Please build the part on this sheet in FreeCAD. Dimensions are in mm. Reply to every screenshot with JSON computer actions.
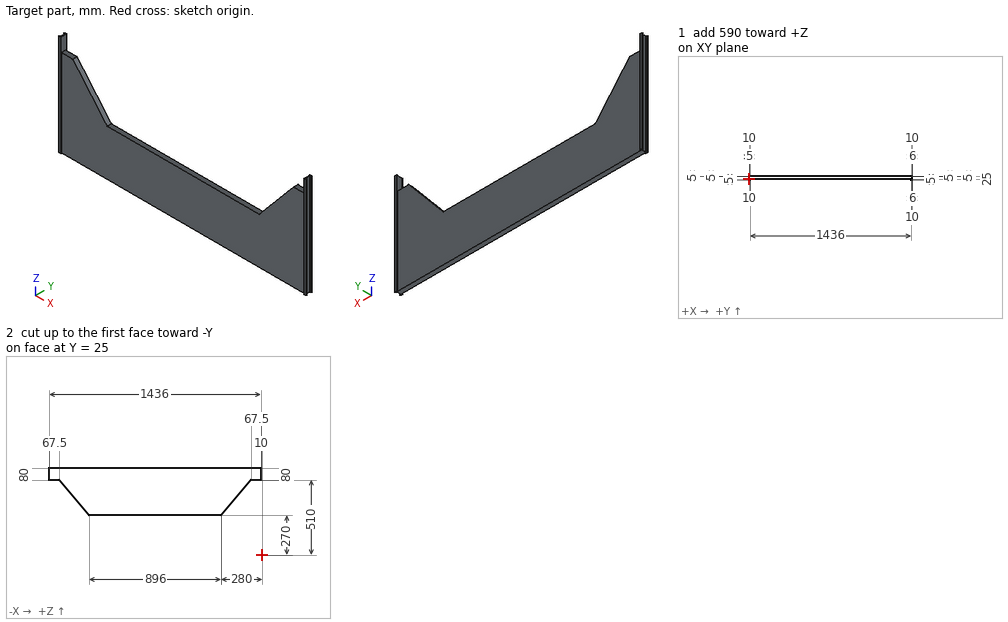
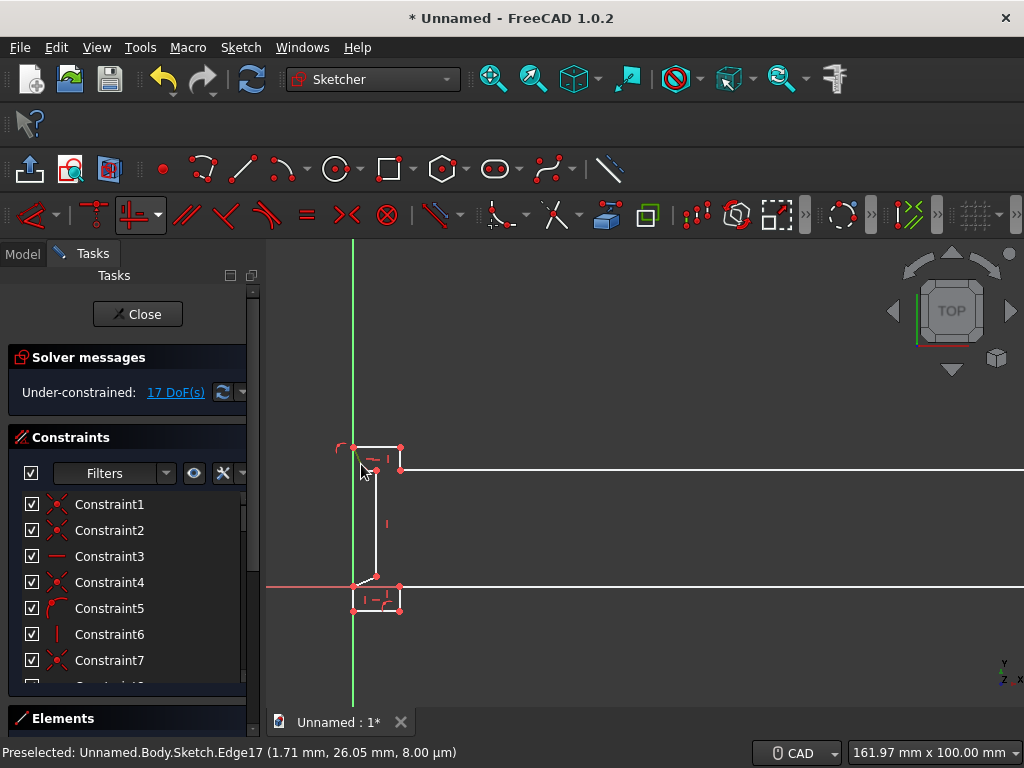
{"action": "key", "text": "v"}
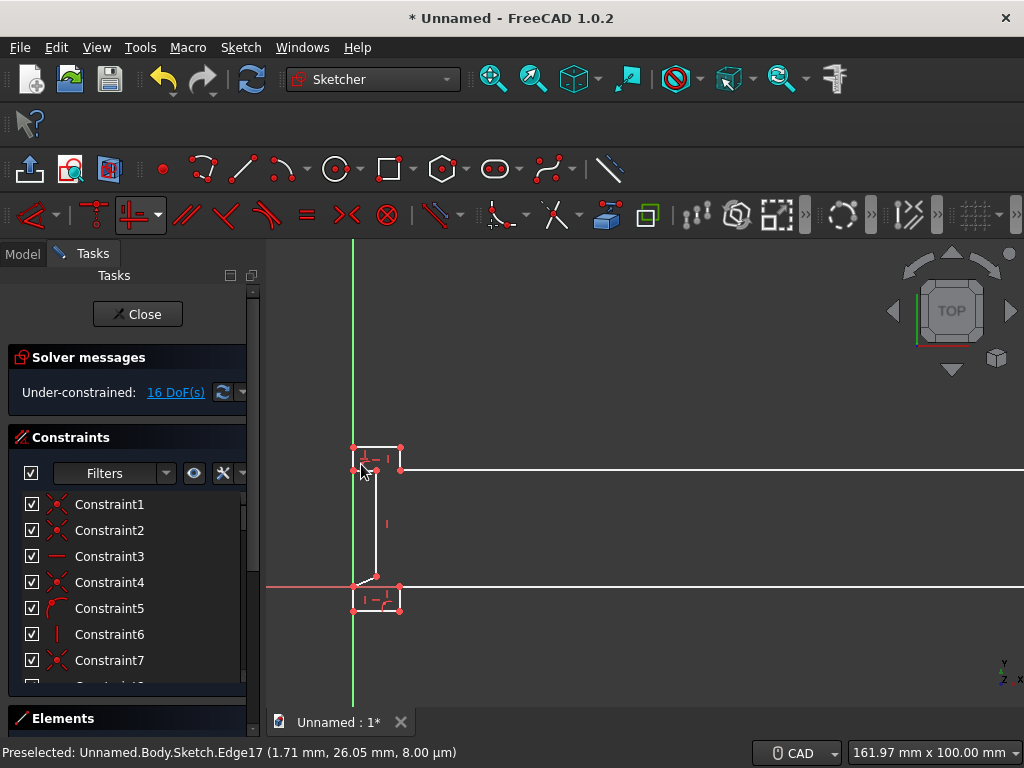
{"action": "left_click", "coordinate": [363, 583]}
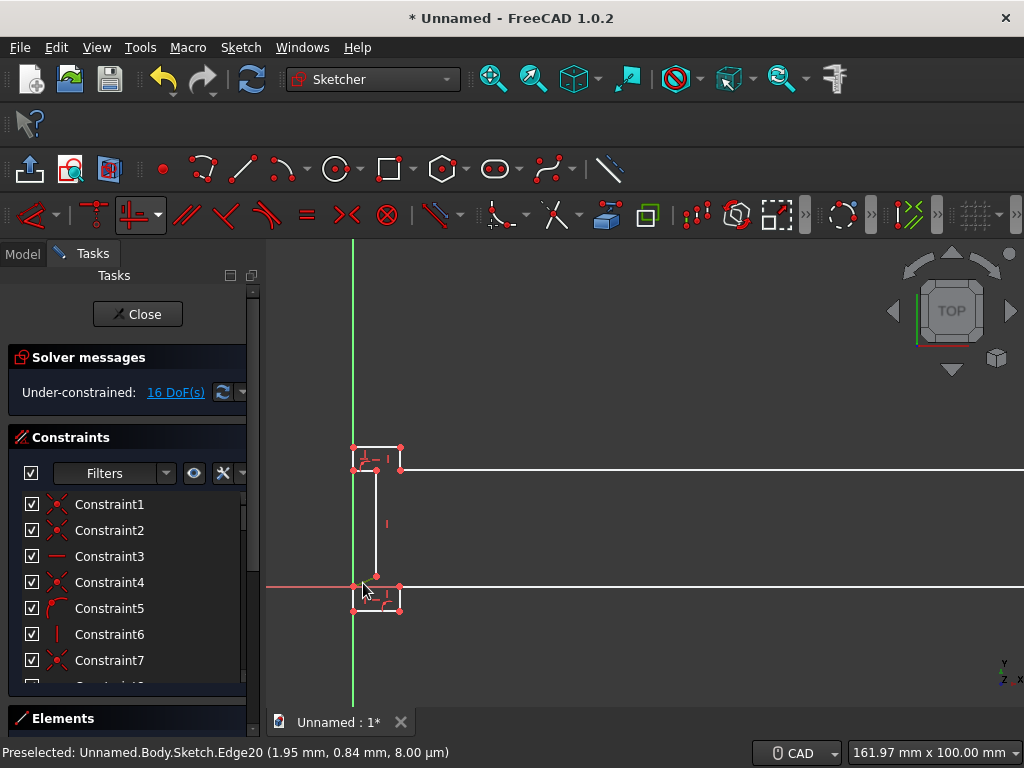
{"action": "key", "text": "h"}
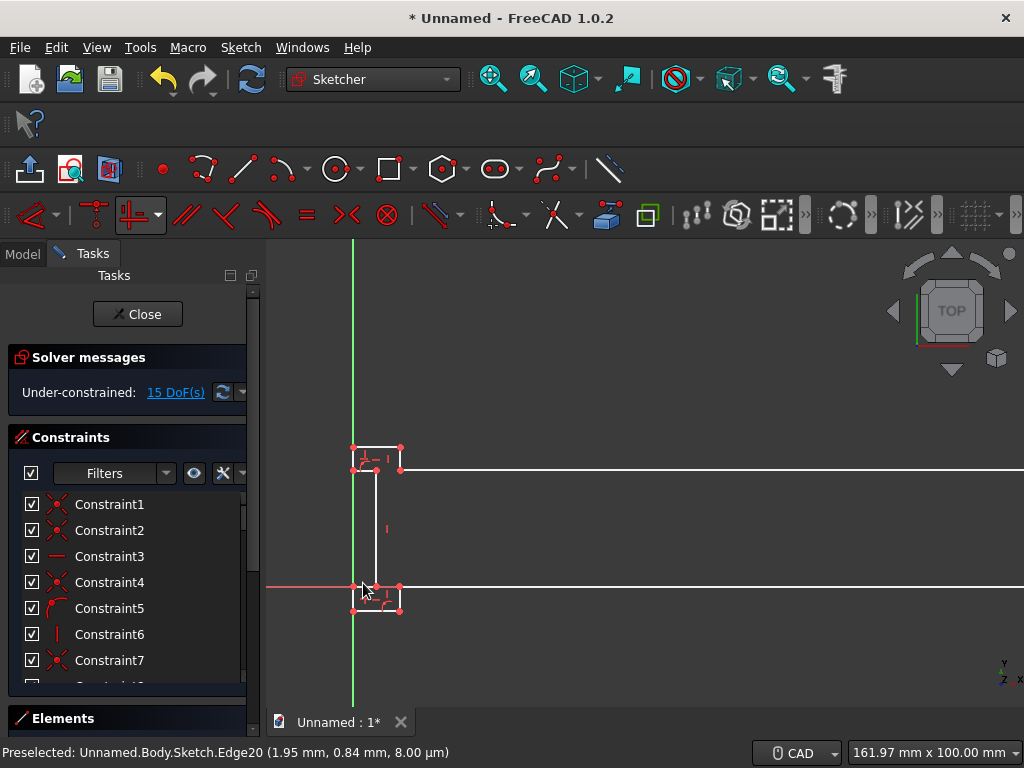
{"action": "key", "text": "d"}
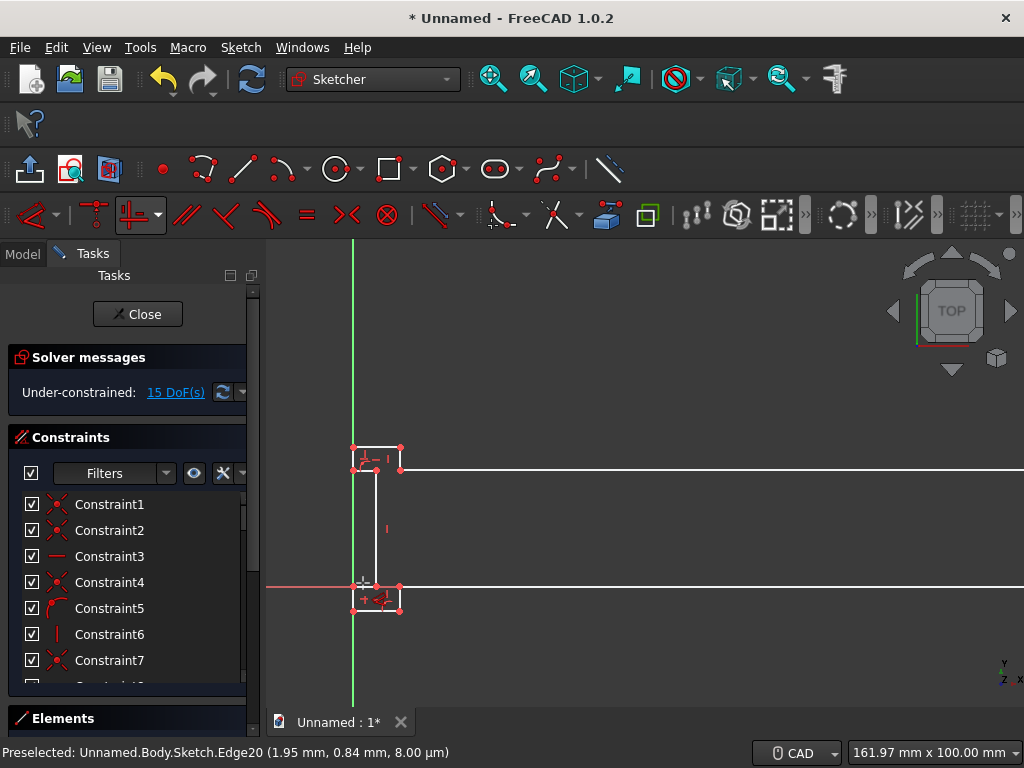
{"action": "scroll", "coordinate": [353, 597], "scroll_direction": "up", "scroll_amount": 3}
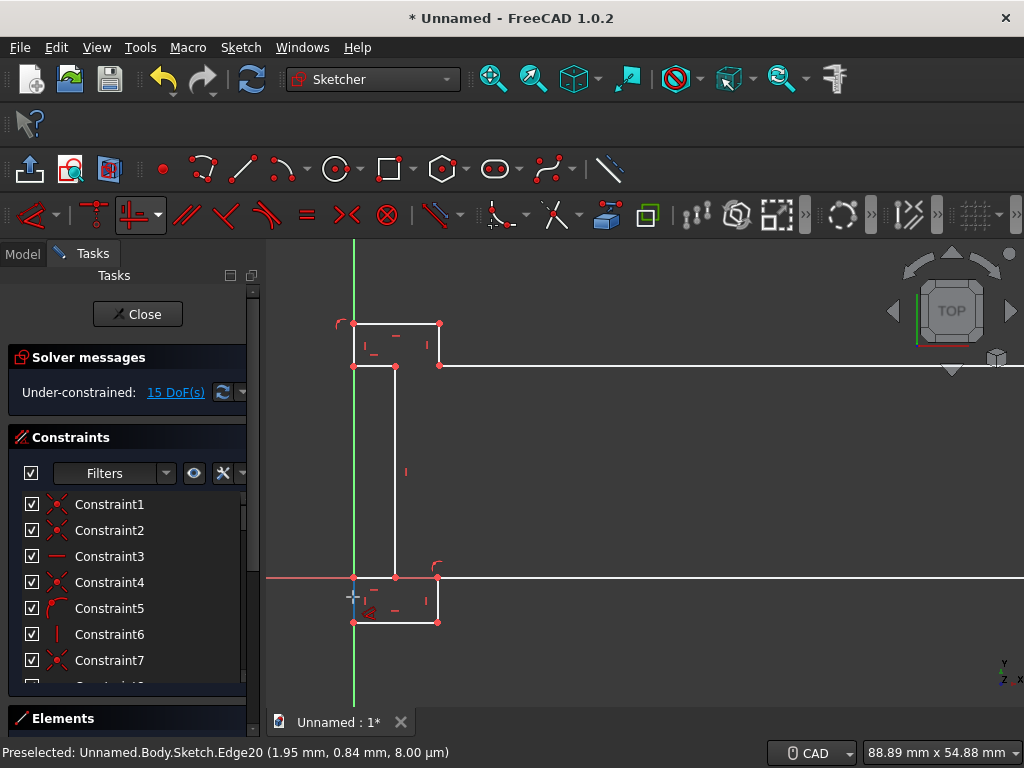
{"action": "left_click", "coordinate": [354, 596]}
{"action": "left_click", "coordinate": [320, 600]}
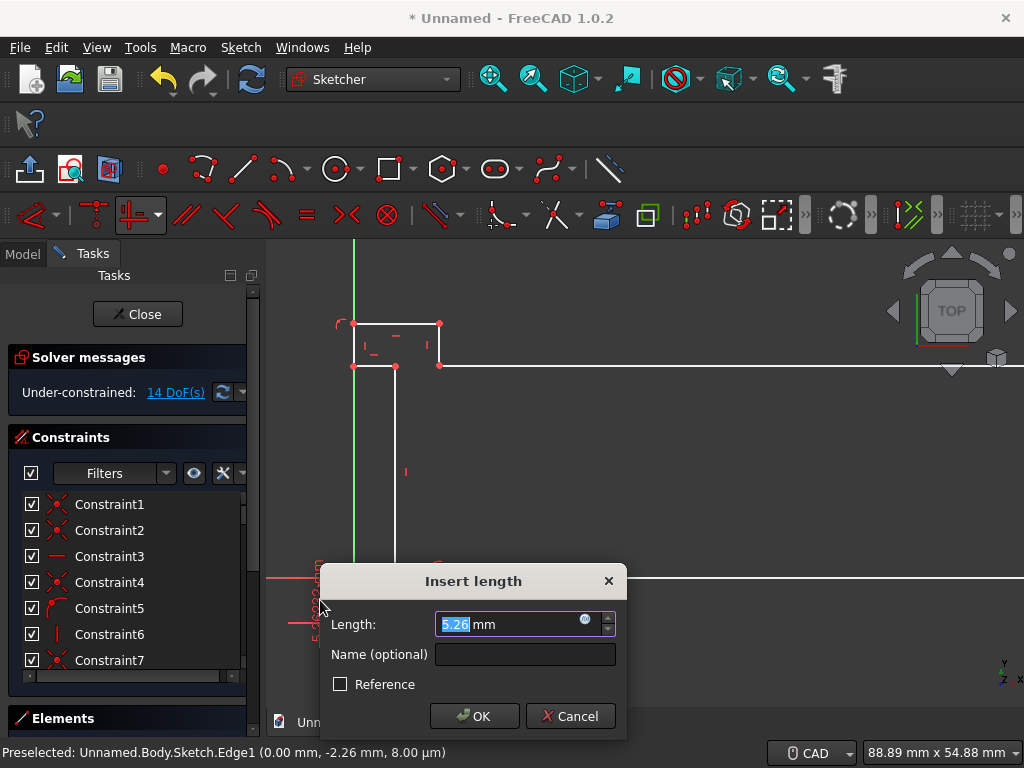
{"action": "type", "text": "5"}
{"action": "key", "text": "Return"}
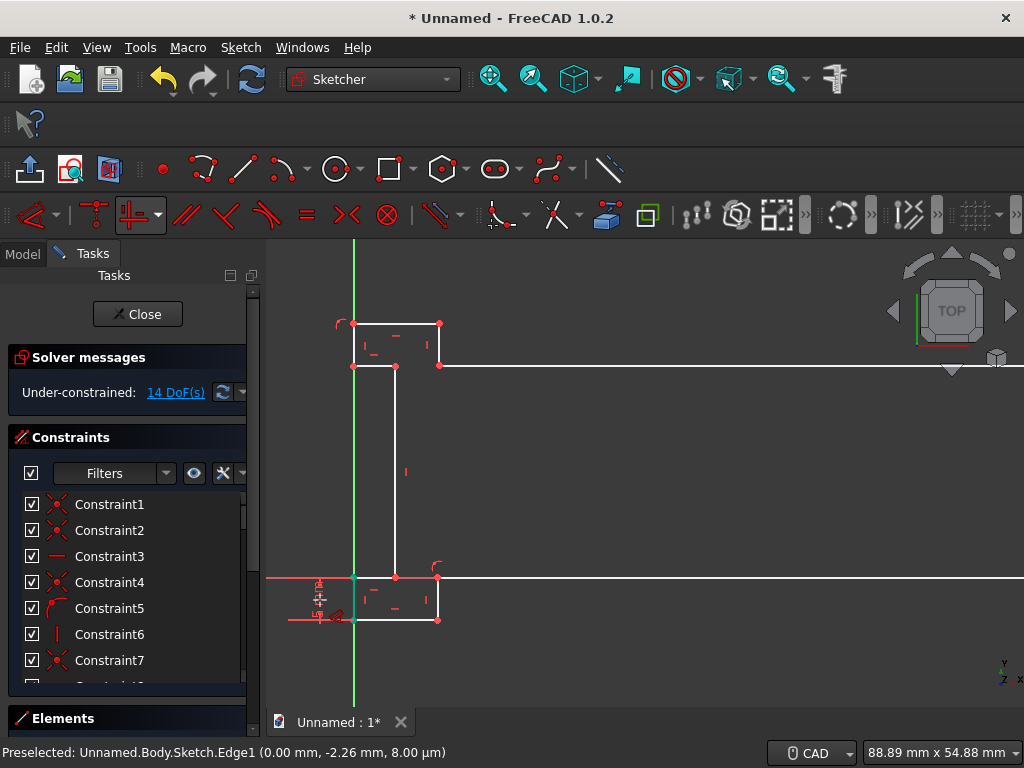
{"action": "scroll", "coordinate": [322, 473], "scroll_direction": "down", "scroll_amount": 16}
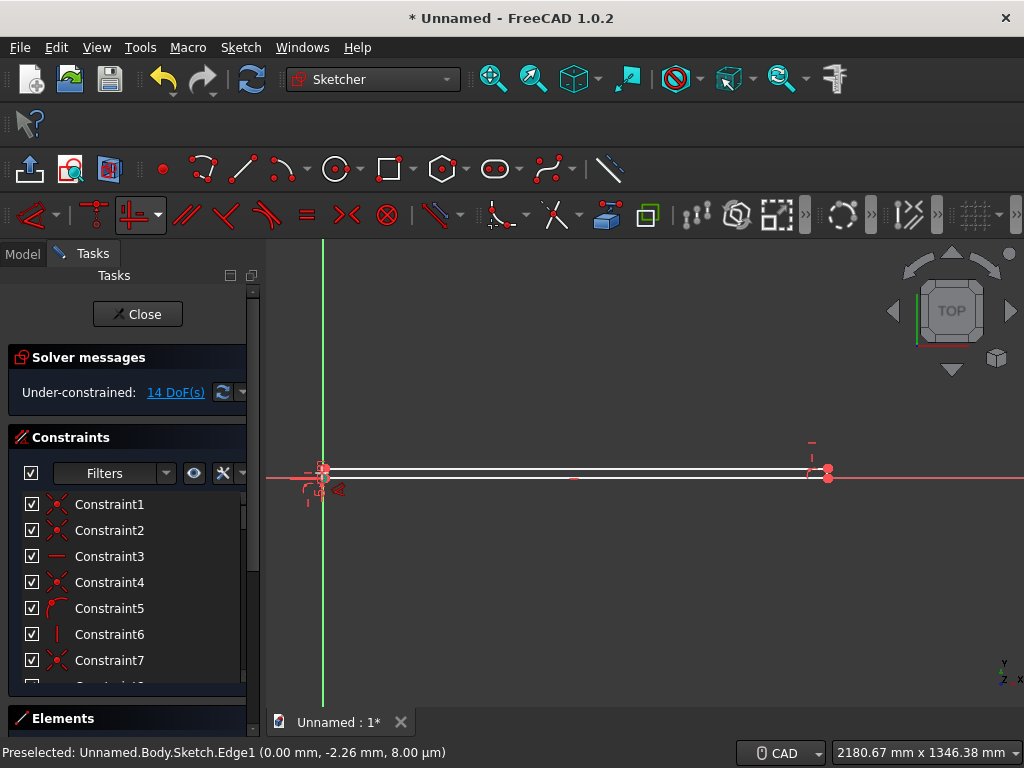
{"action": "scroll", "coordinate": [827, 478], "scroll_direction": "up", "scroll_amount": 16}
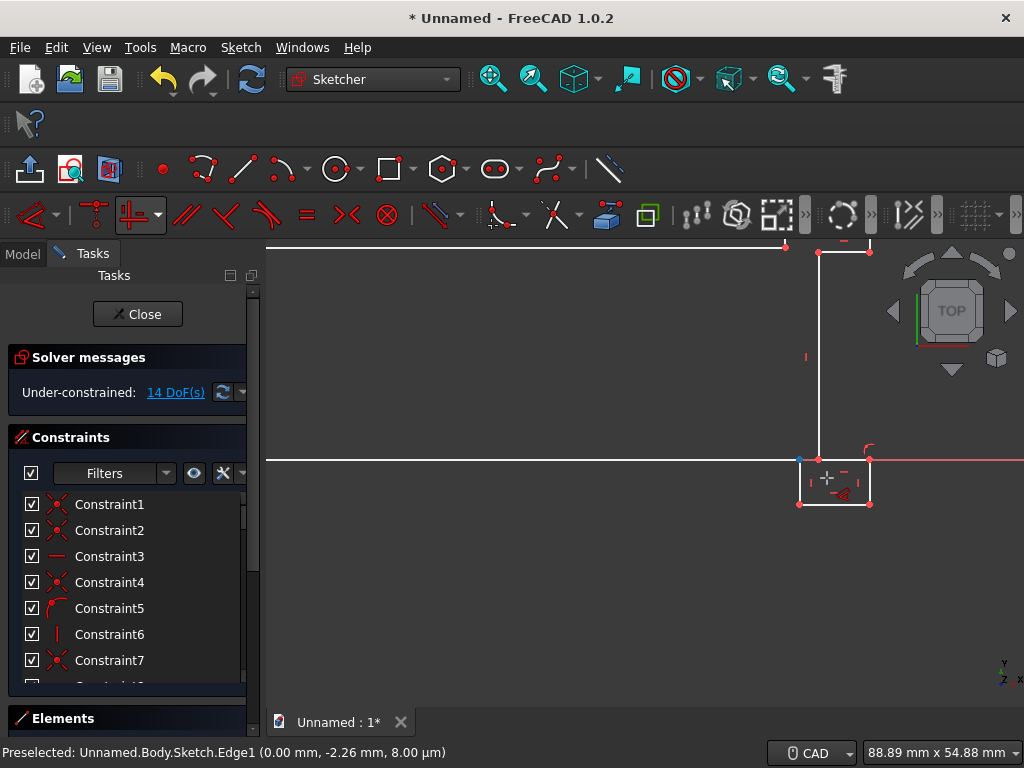
{"action": "left_click", "coordinate": [800, 473]}
{"action": "left_click", "coordinate": [834, 482]}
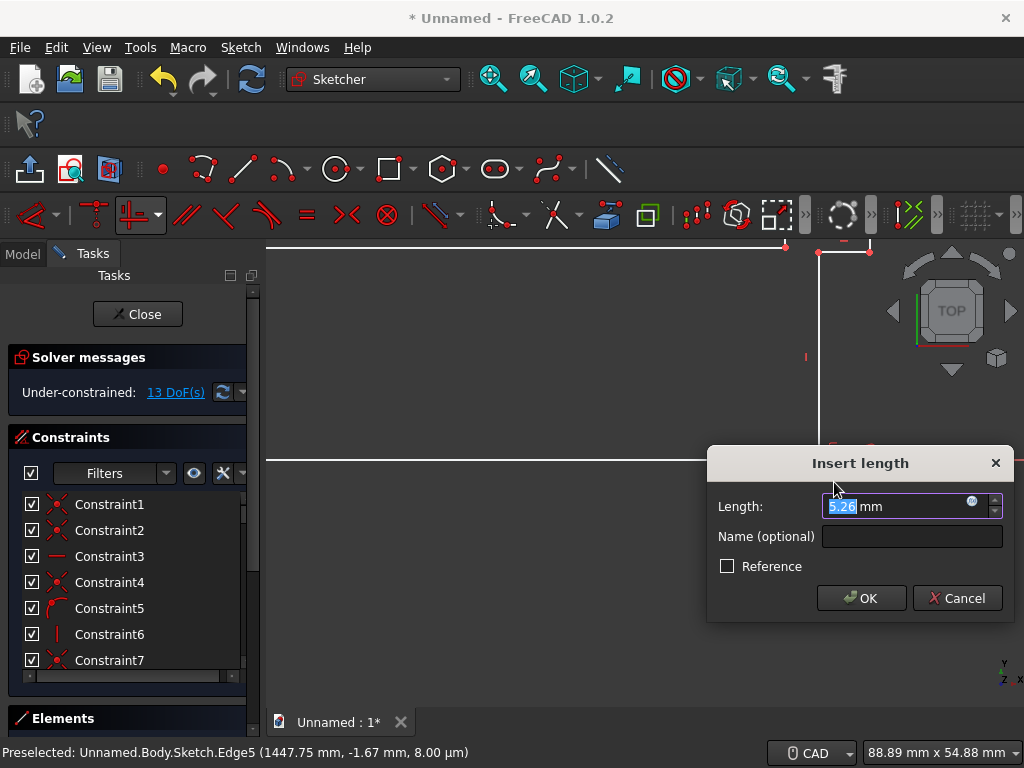
{"action": "type", "text": "5"}
{"action": "key", "text": "Return"}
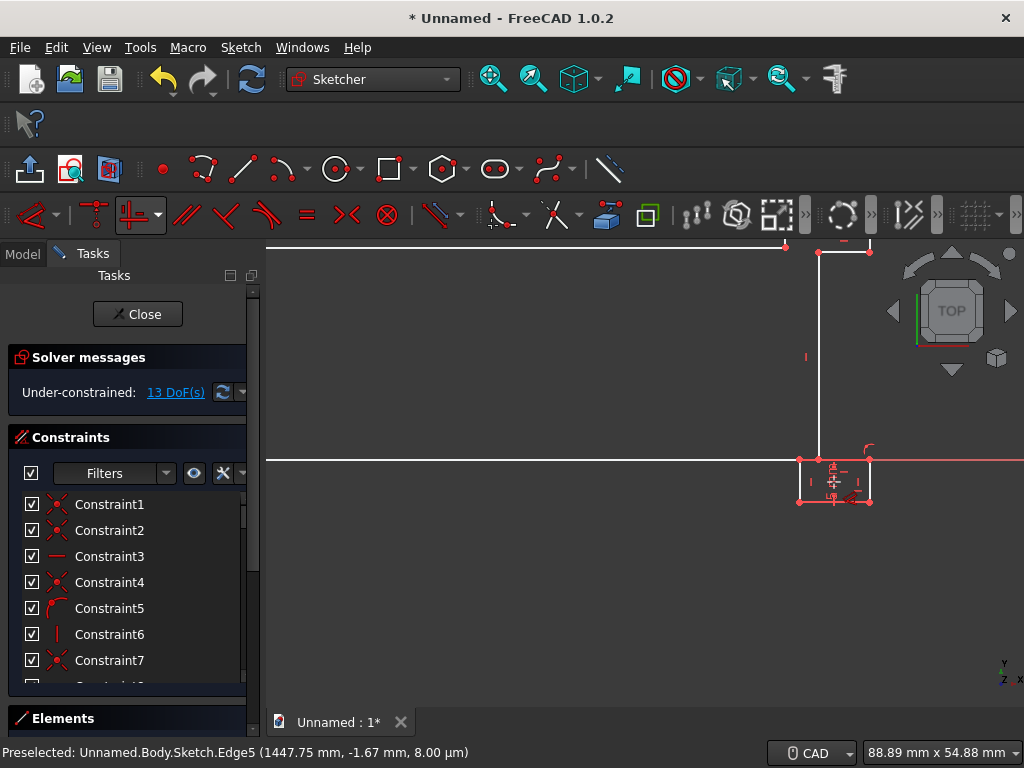
{"action": "left_click", "coordinate": [854, 460]}
{"action": "left_click", "coordinate": [839, 426]}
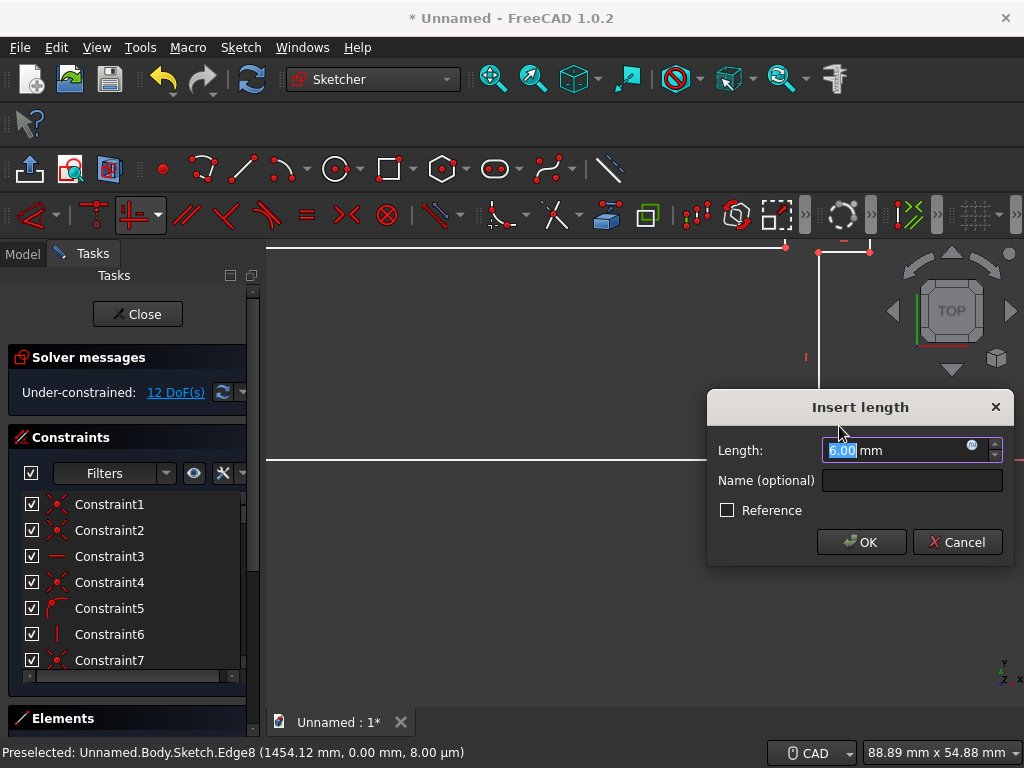
{"action": "type", "text": "6"}
{"action": "key", "text": "Return"}